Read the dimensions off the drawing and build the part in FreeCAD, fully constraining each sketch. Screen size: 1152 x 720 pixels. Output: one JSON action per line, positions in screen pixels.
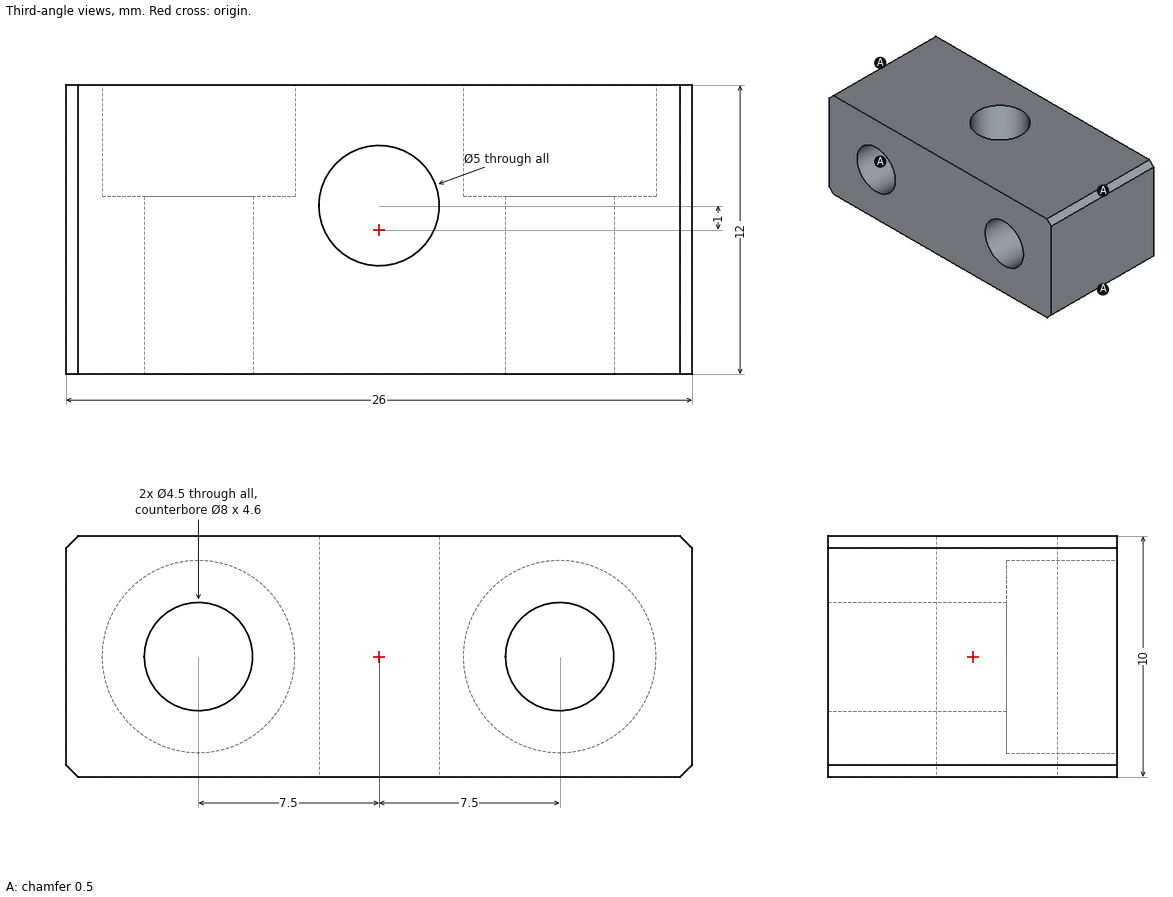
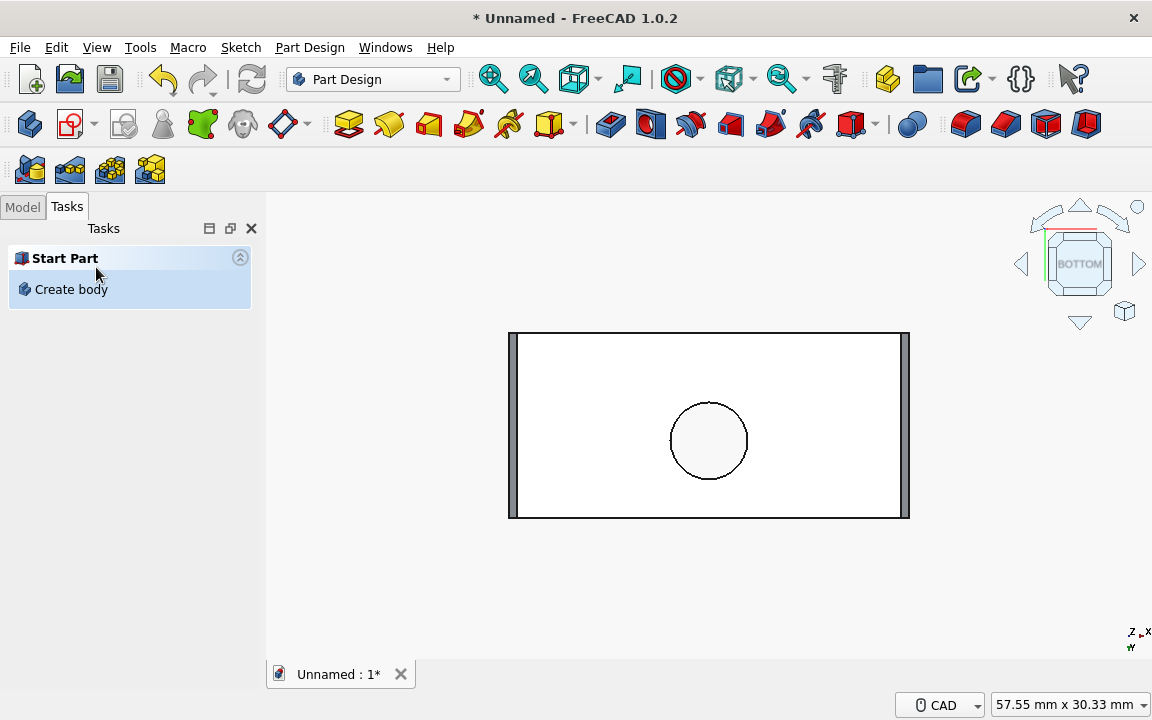
{"action": "key", "text": "0"}